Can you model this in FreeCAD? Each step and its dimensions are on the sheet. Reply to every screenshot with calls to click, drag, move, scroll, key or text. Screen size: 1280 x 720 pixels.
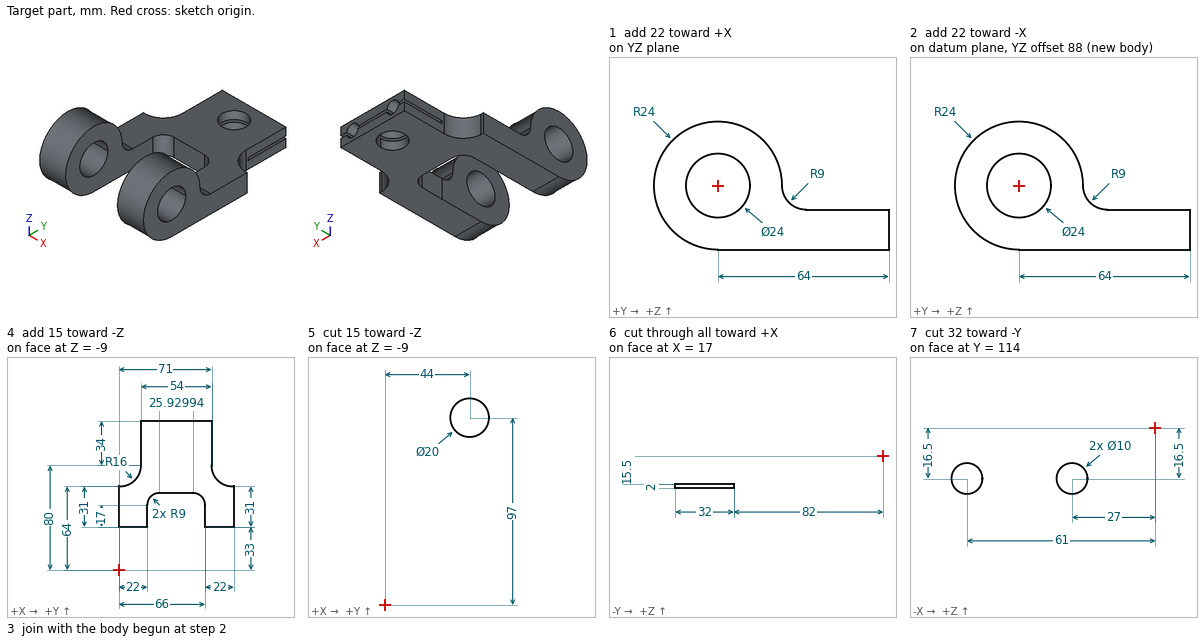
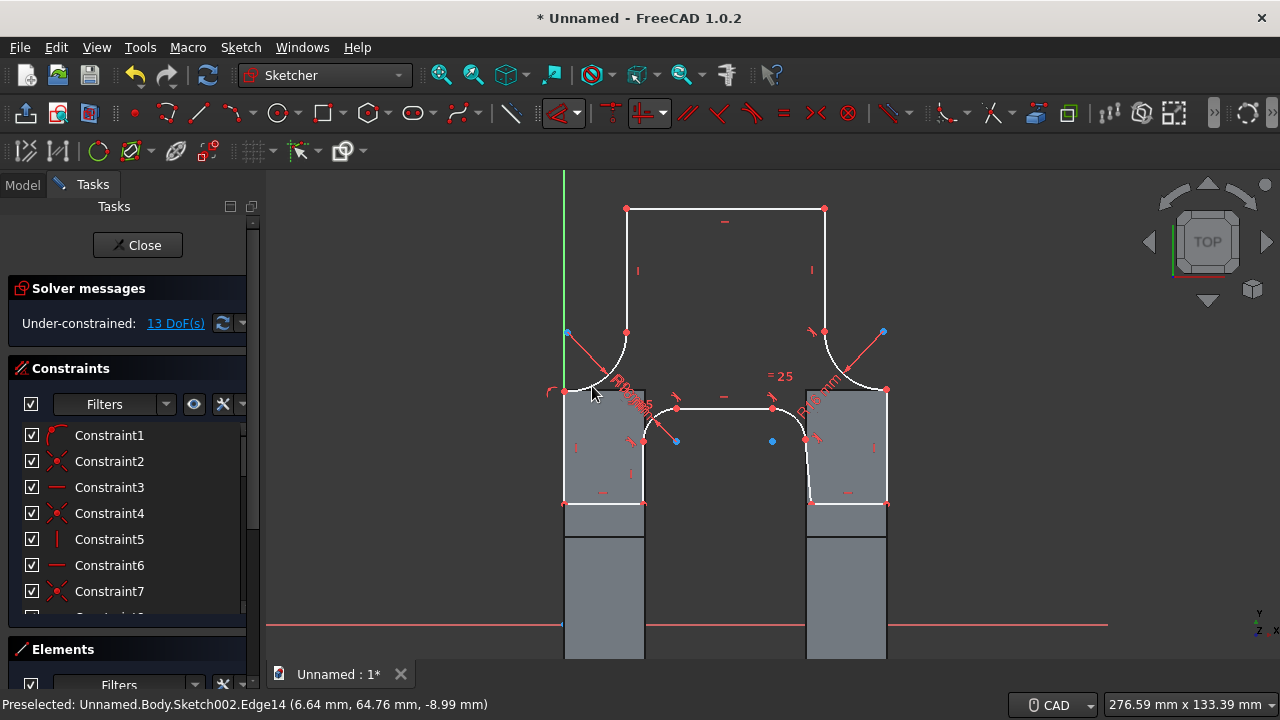
click(564, 425)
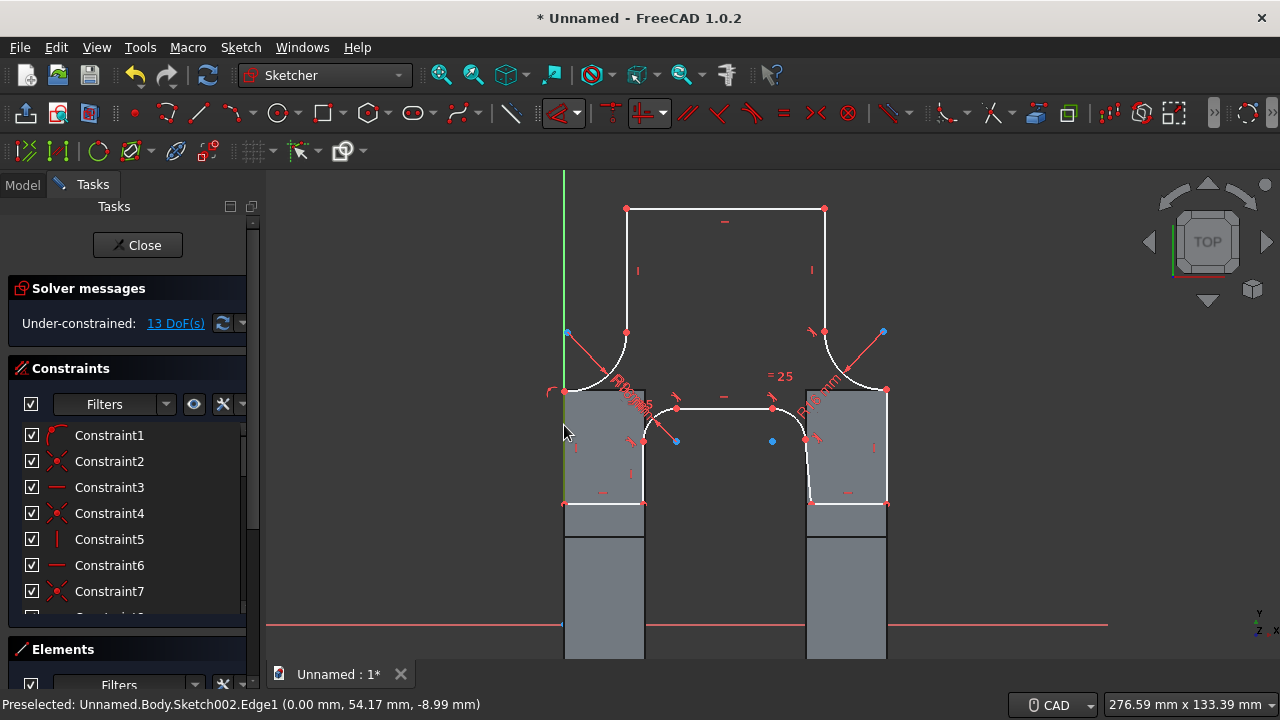
key(i)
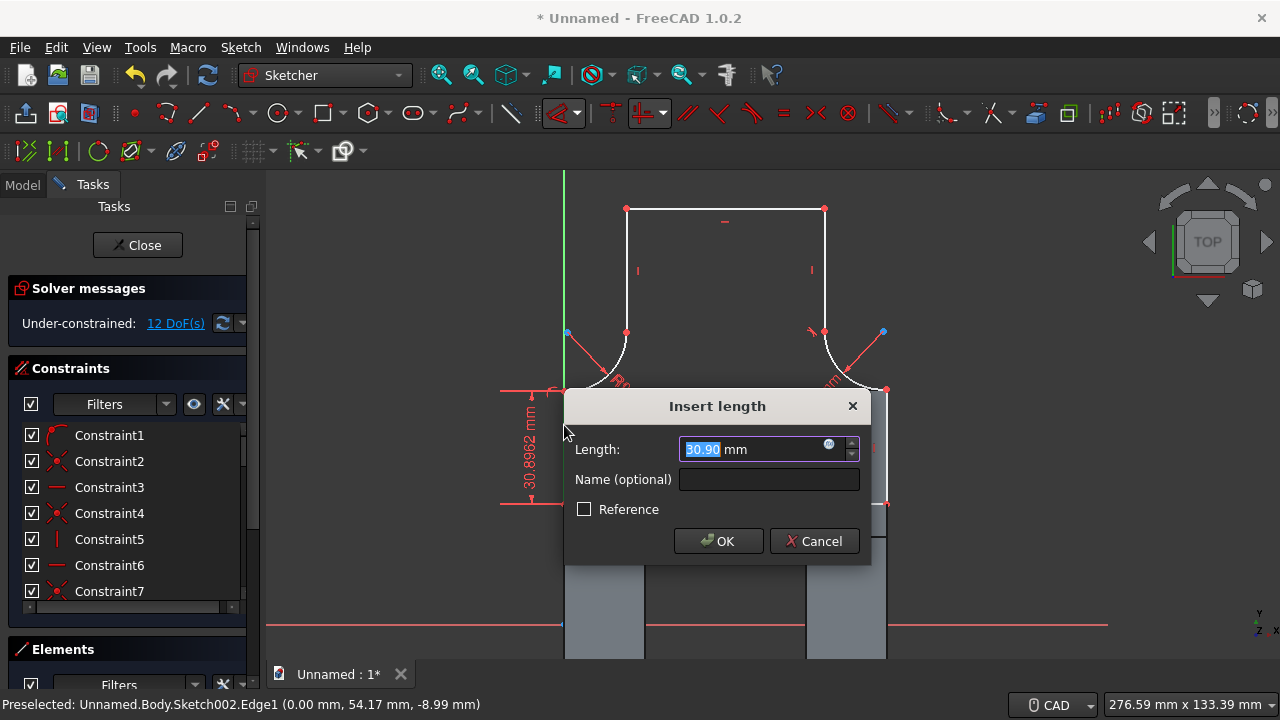
text(31)
key(Return)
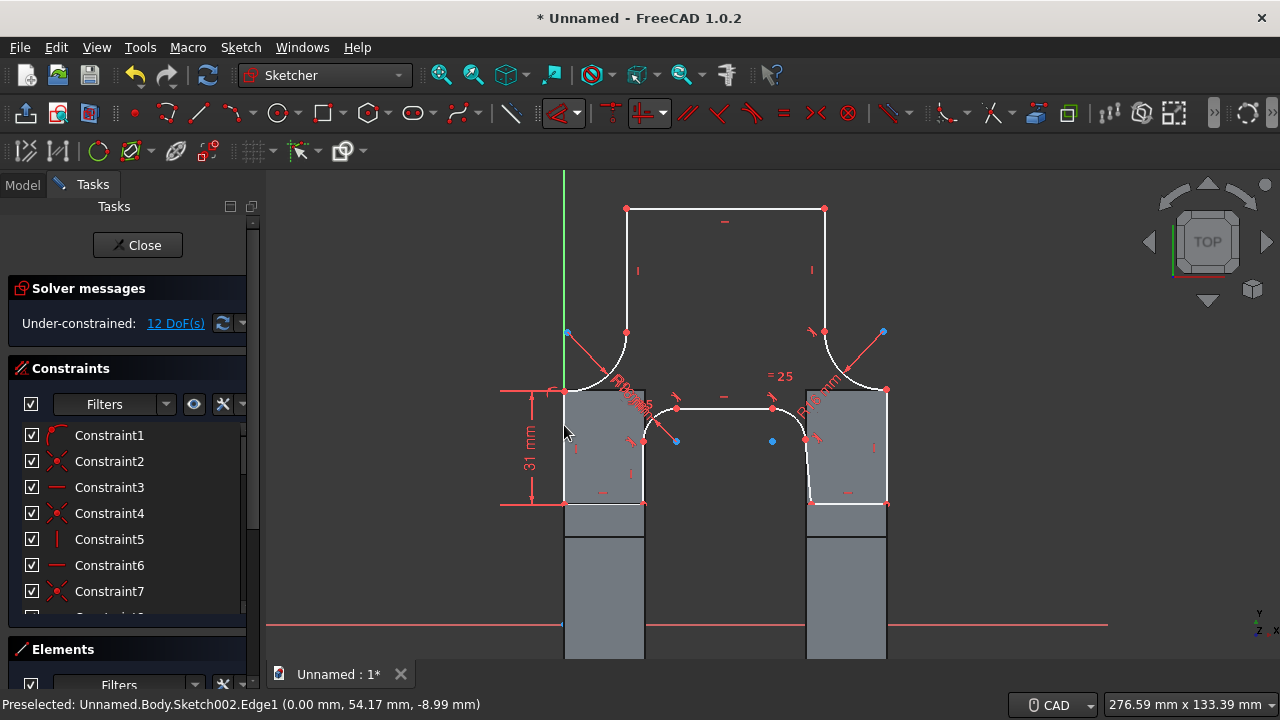
click(588, 505)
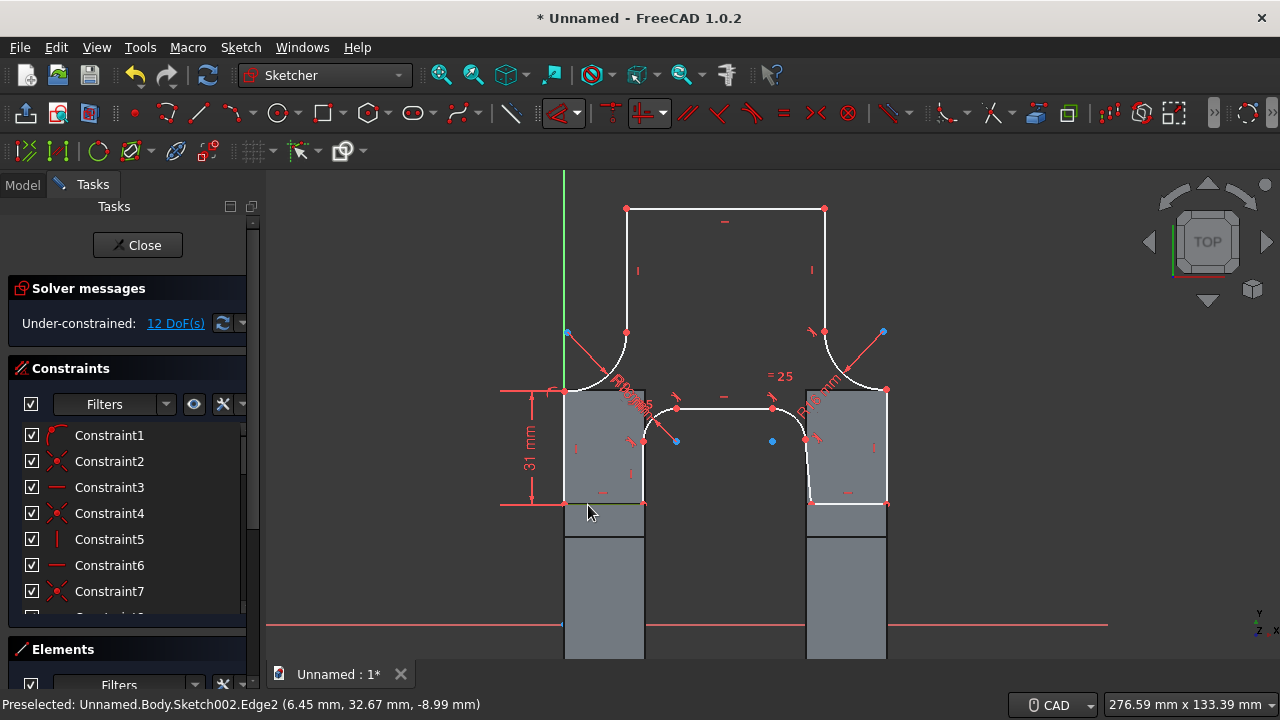
key(l)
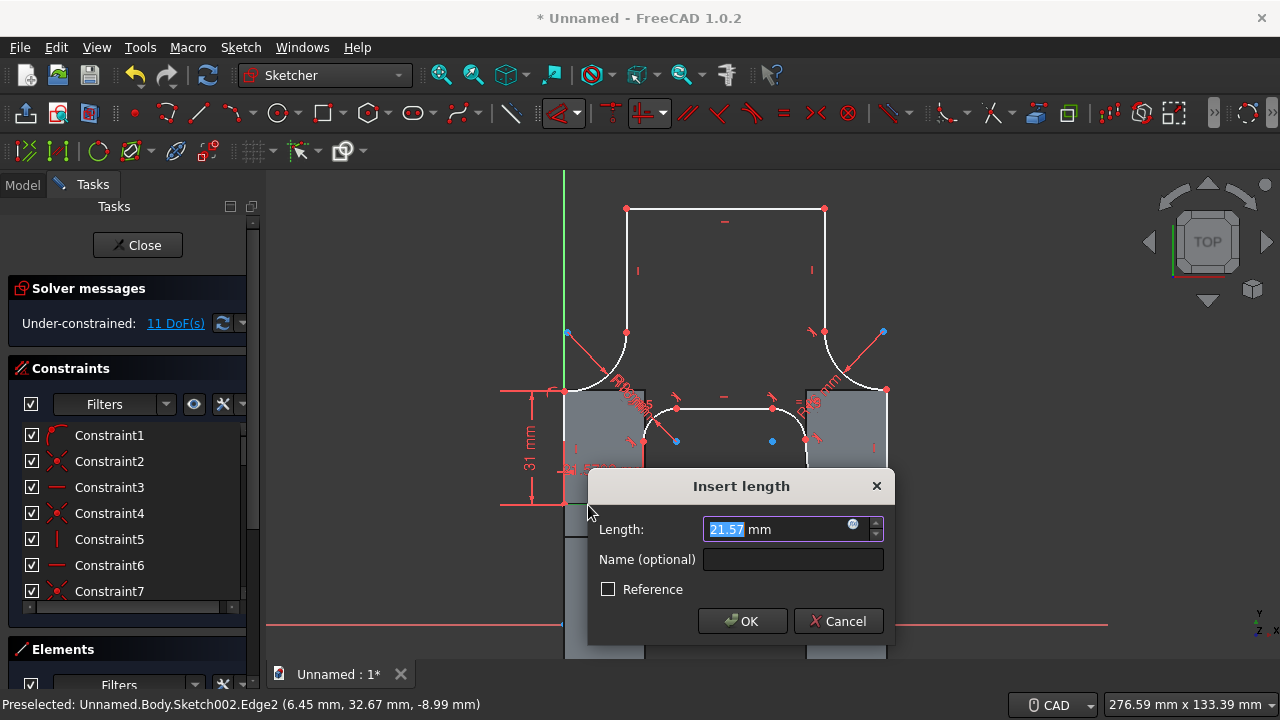
text(22)
key(Return)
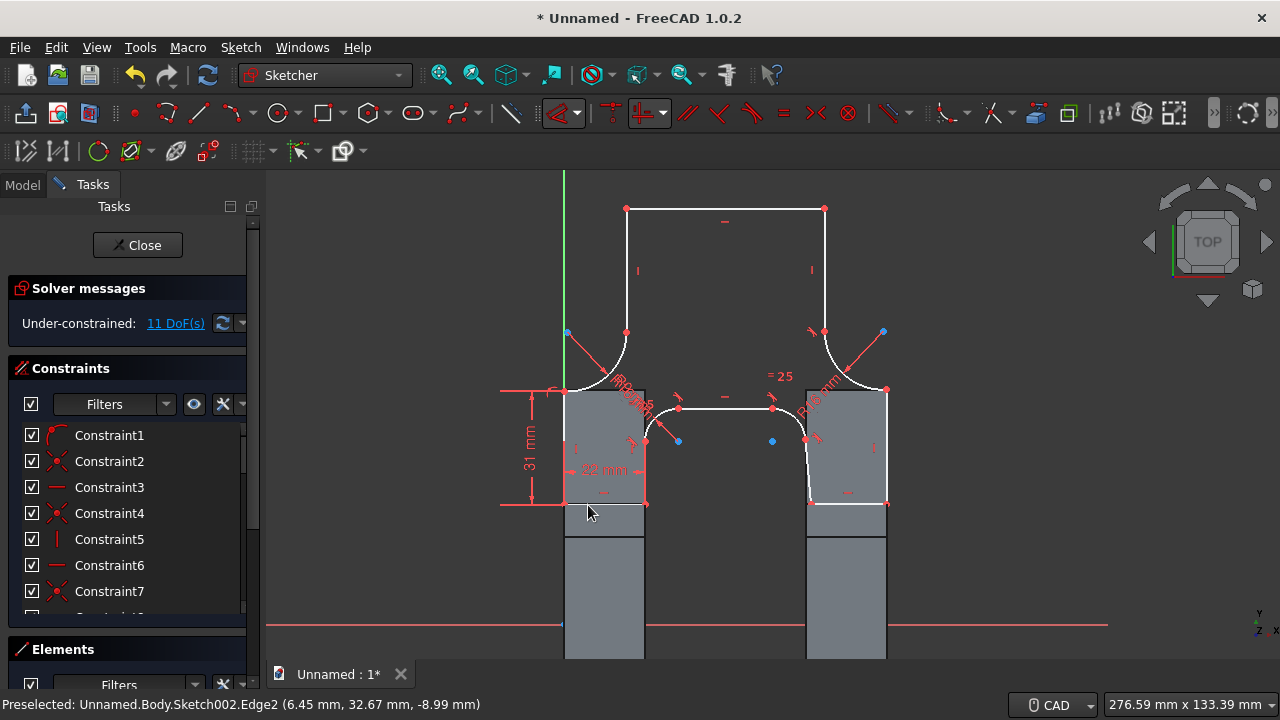
click(645, 486)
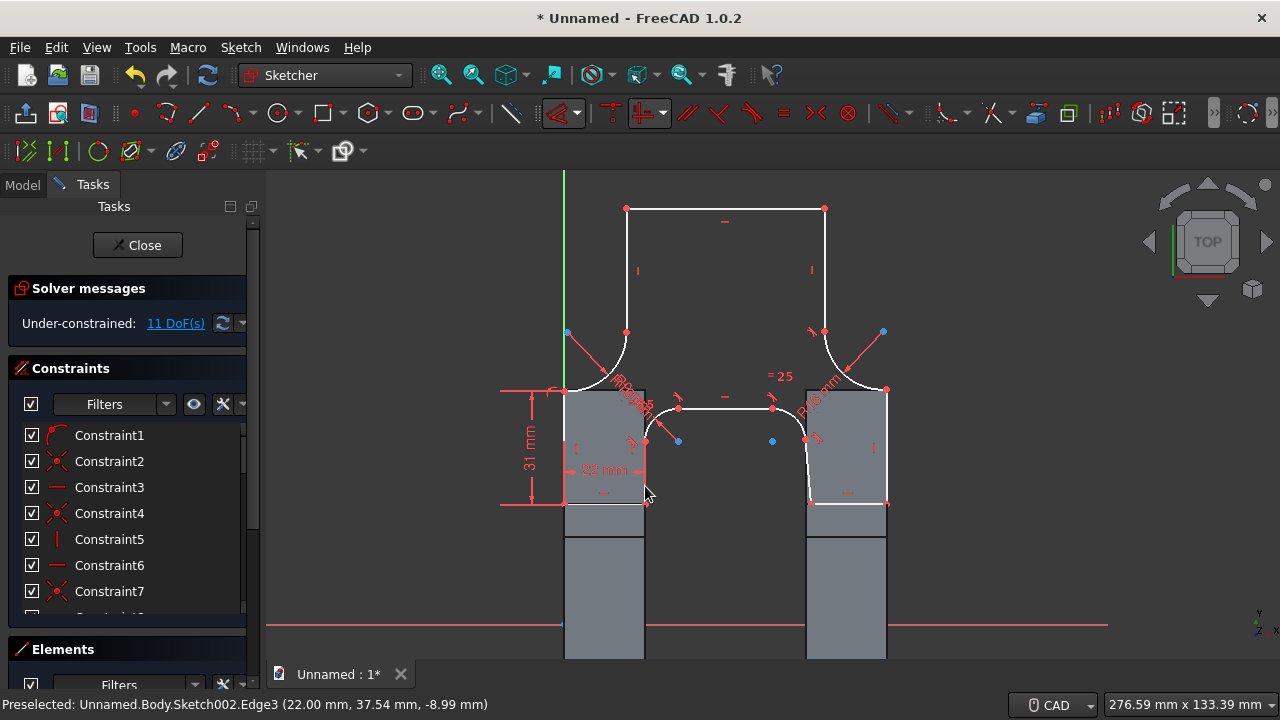
key(i)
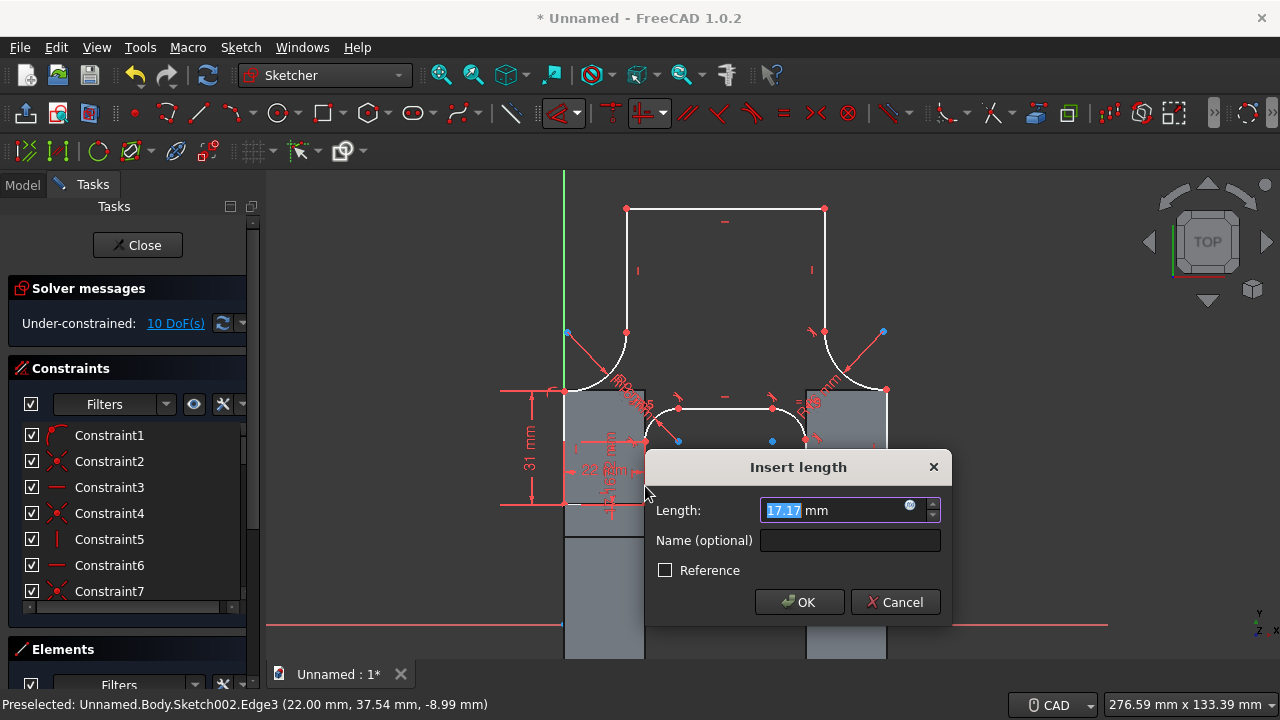
text(17)
key(Return)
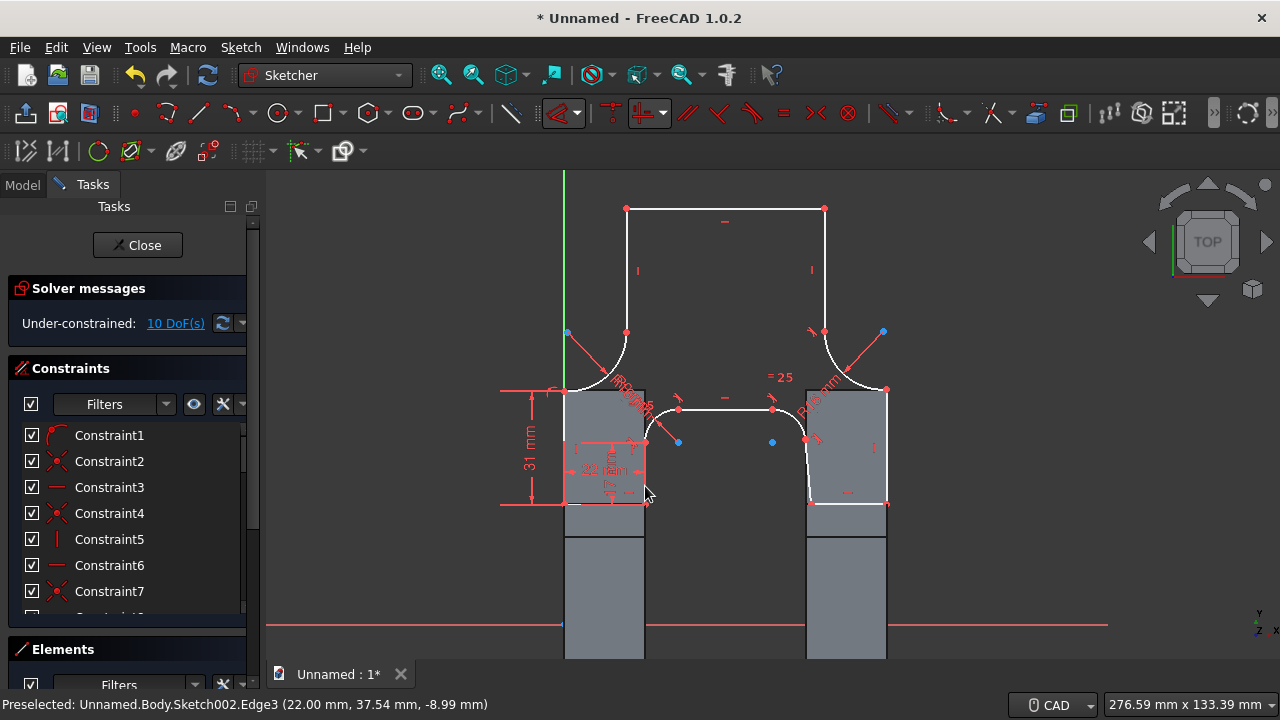
click(834, 504)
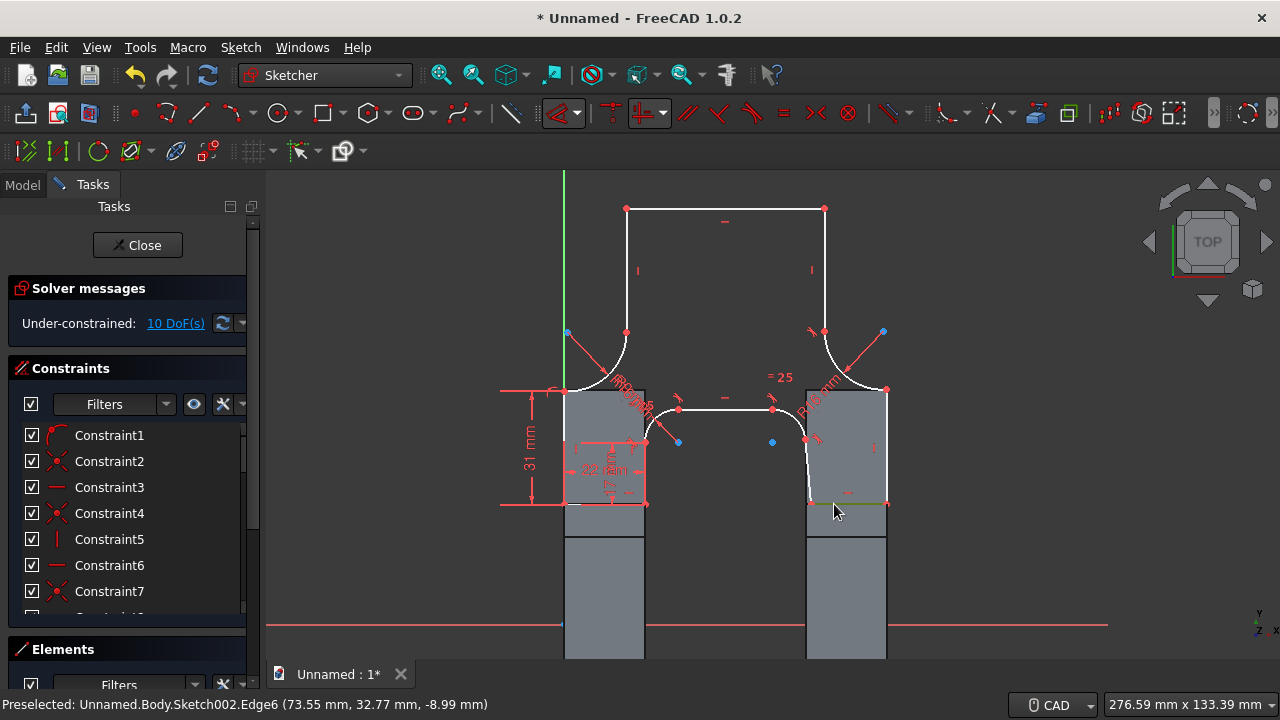
click(580, 114)